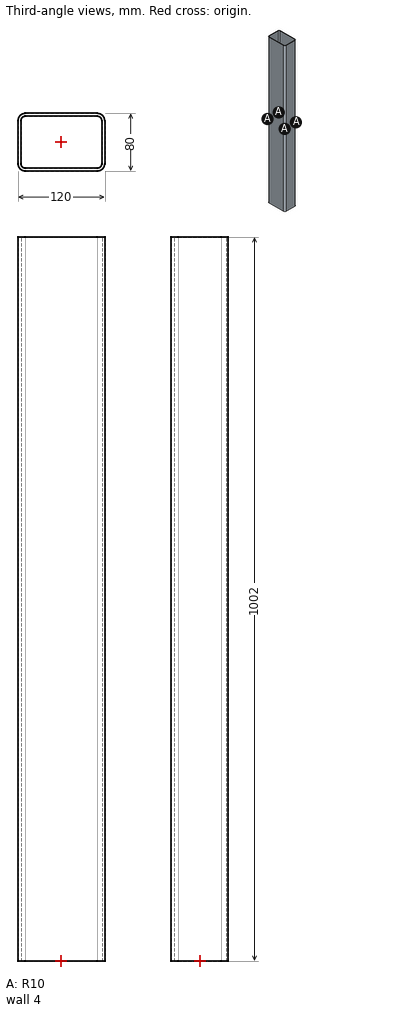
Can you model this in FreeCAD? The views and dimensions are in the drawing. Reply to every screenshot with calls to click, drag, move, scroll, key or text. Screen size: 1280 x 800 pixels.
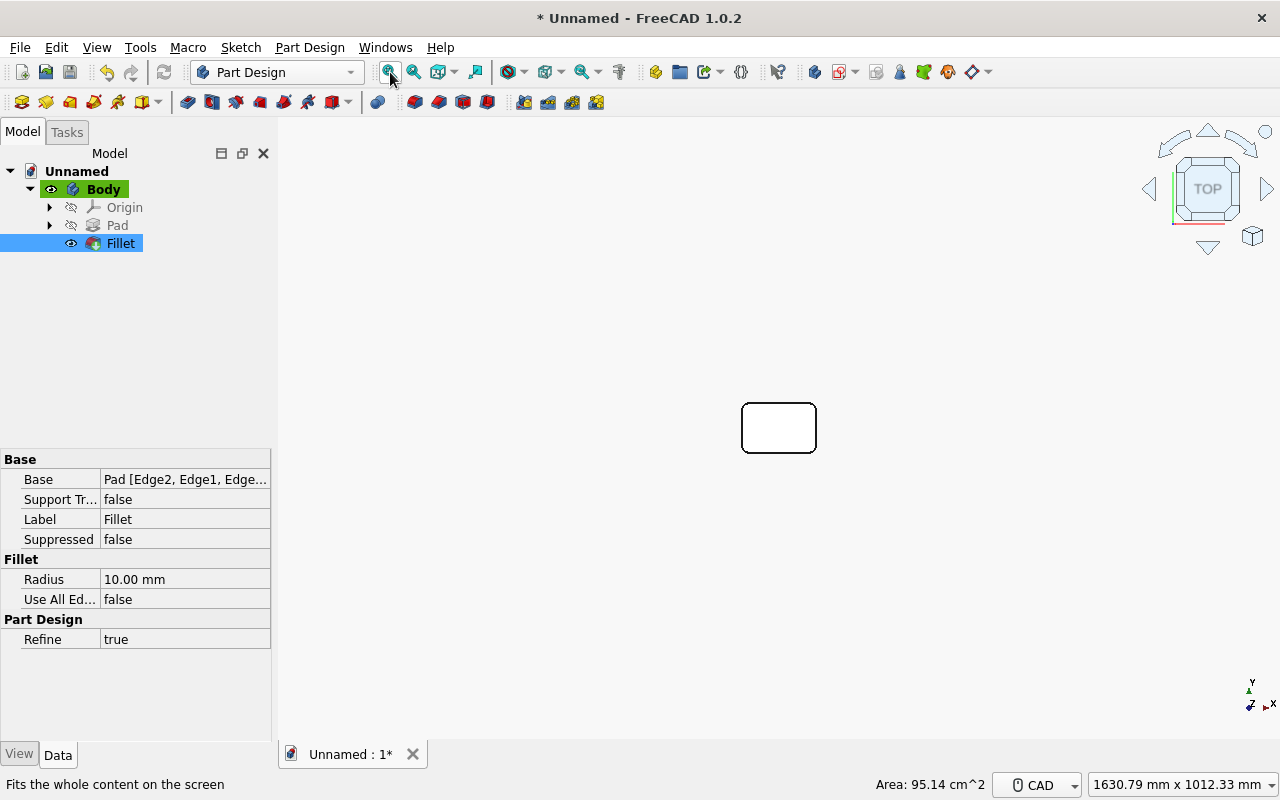
key(1)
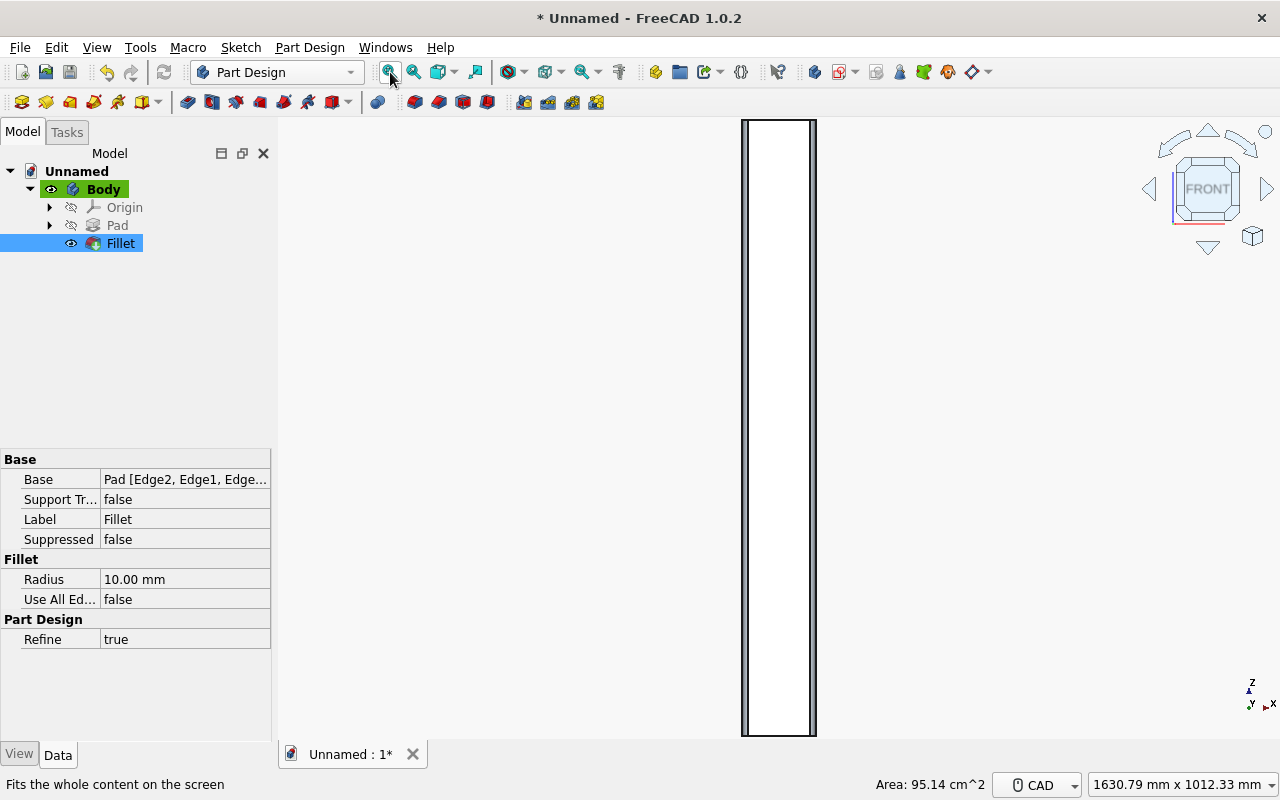
key(3)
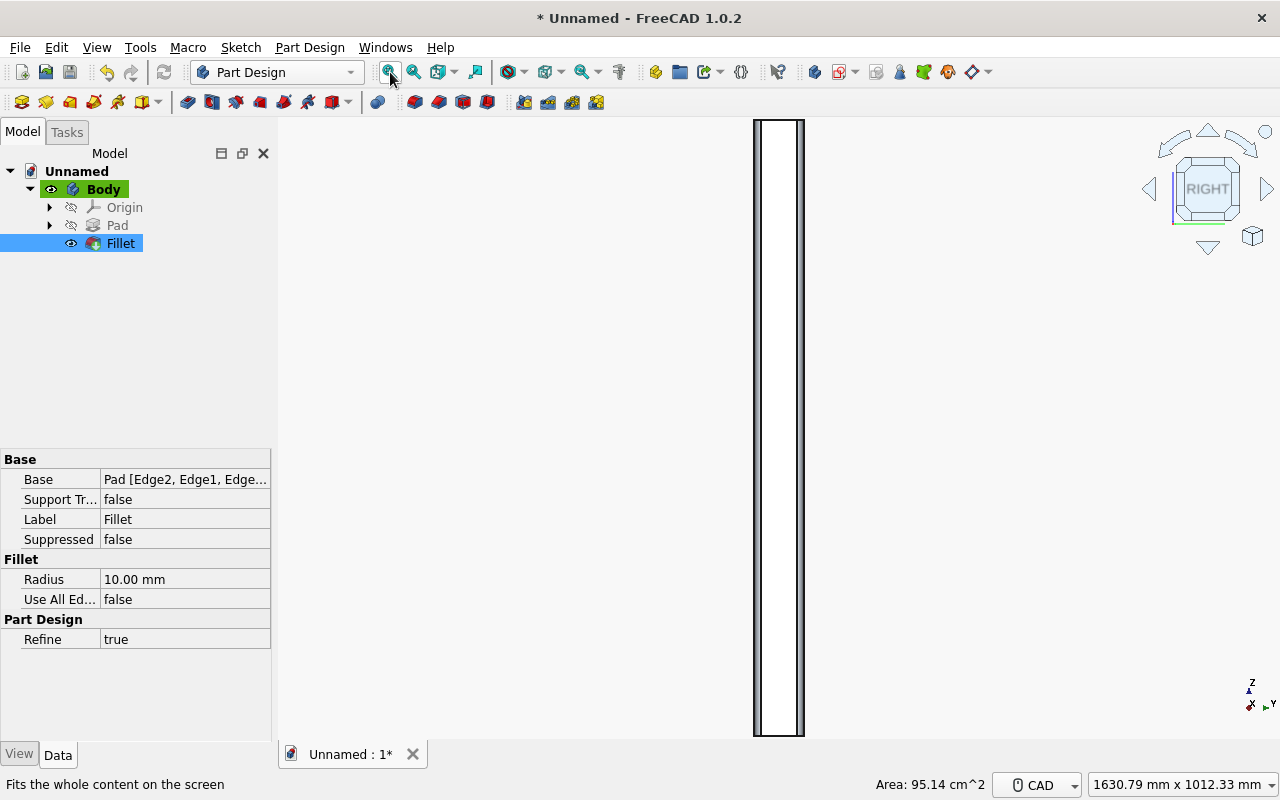
key(5)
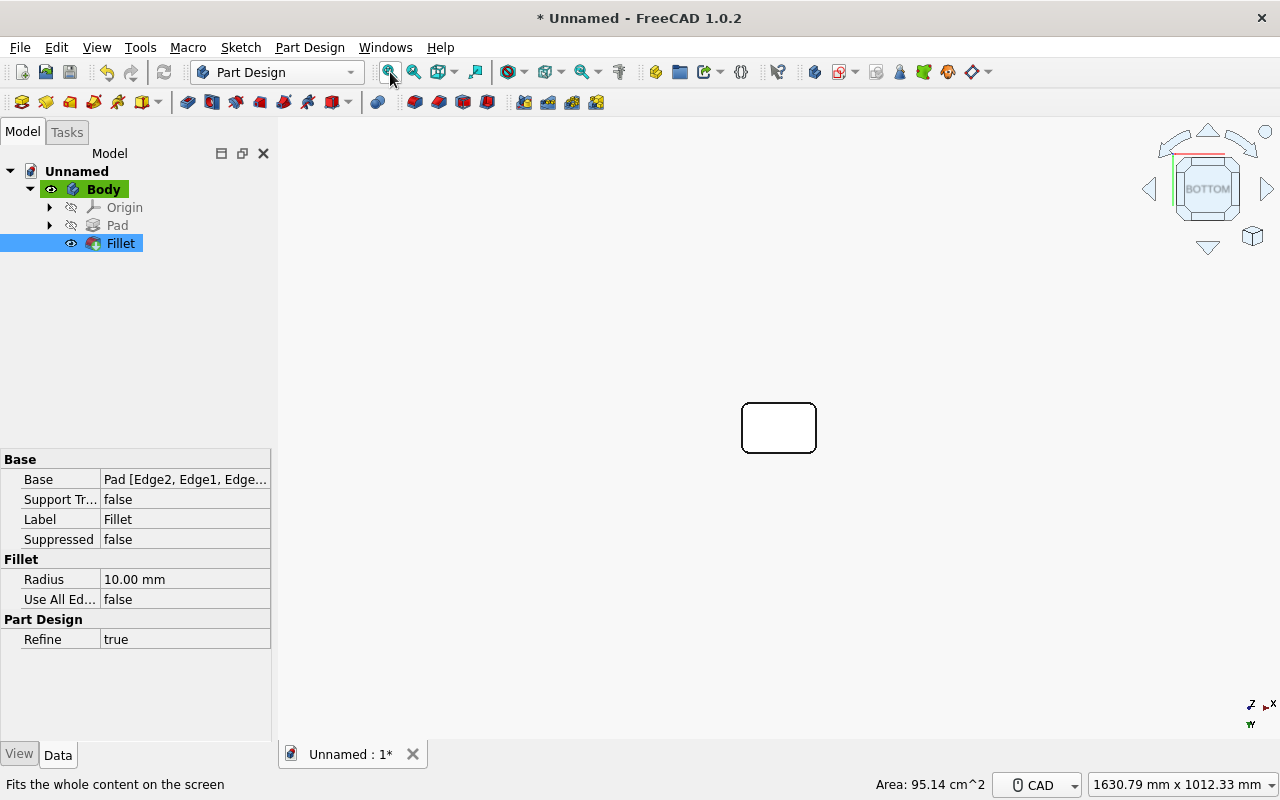
click(390, 72)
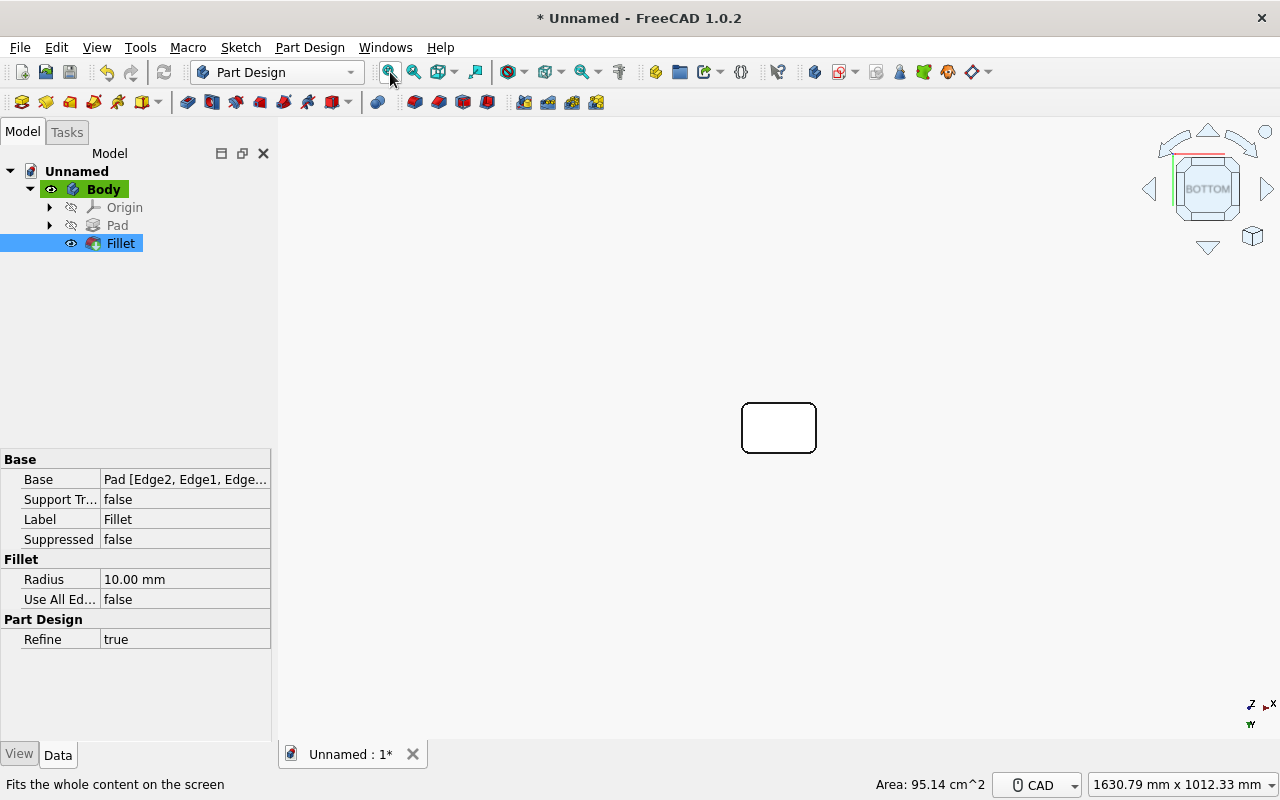
click(790, 427, ctrl)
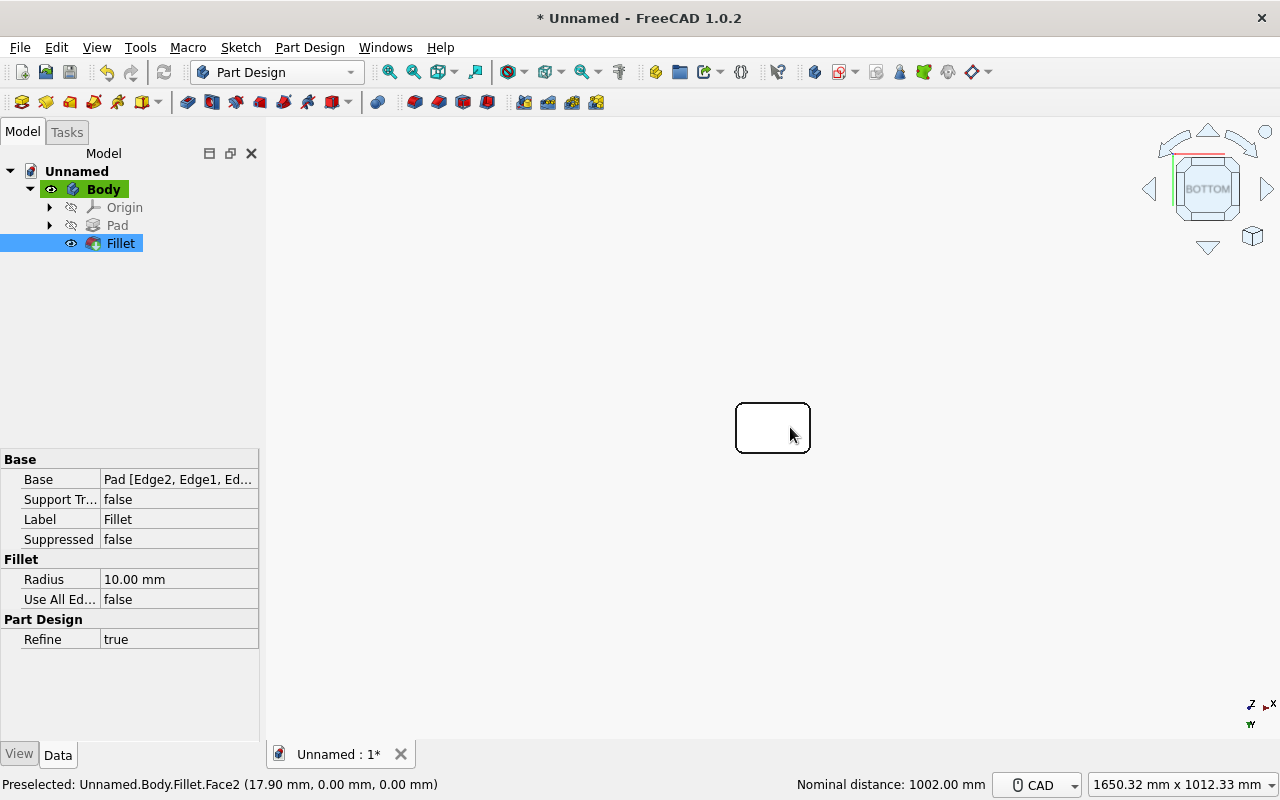
click(488, 102)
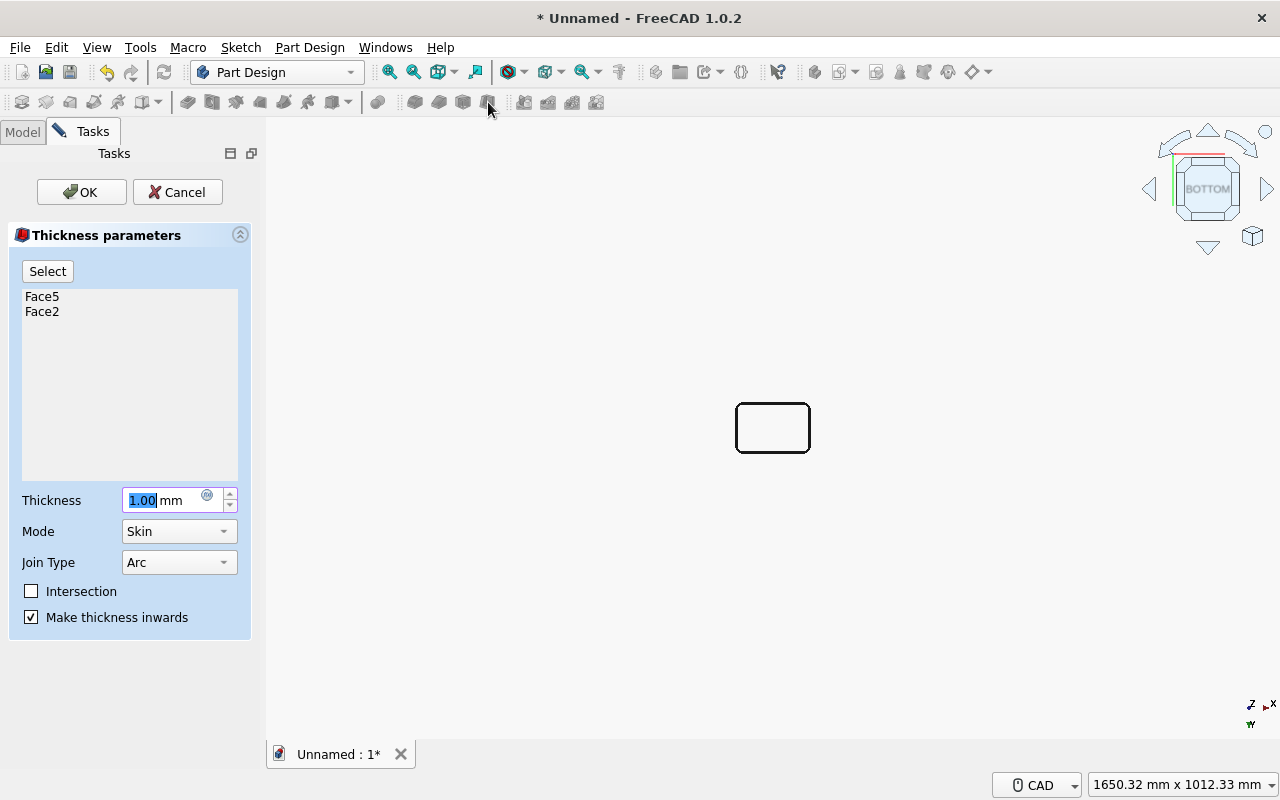
text(4)
key(Tab)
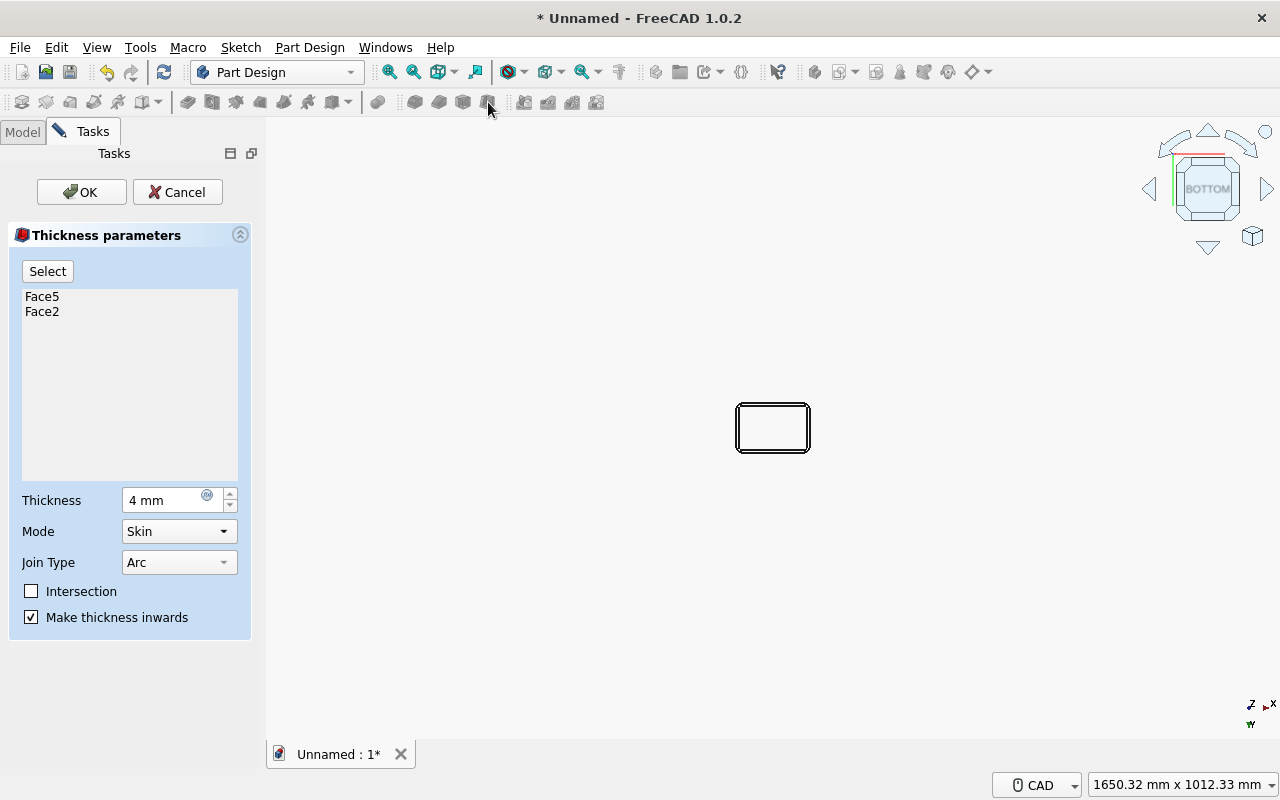
click(180, 562)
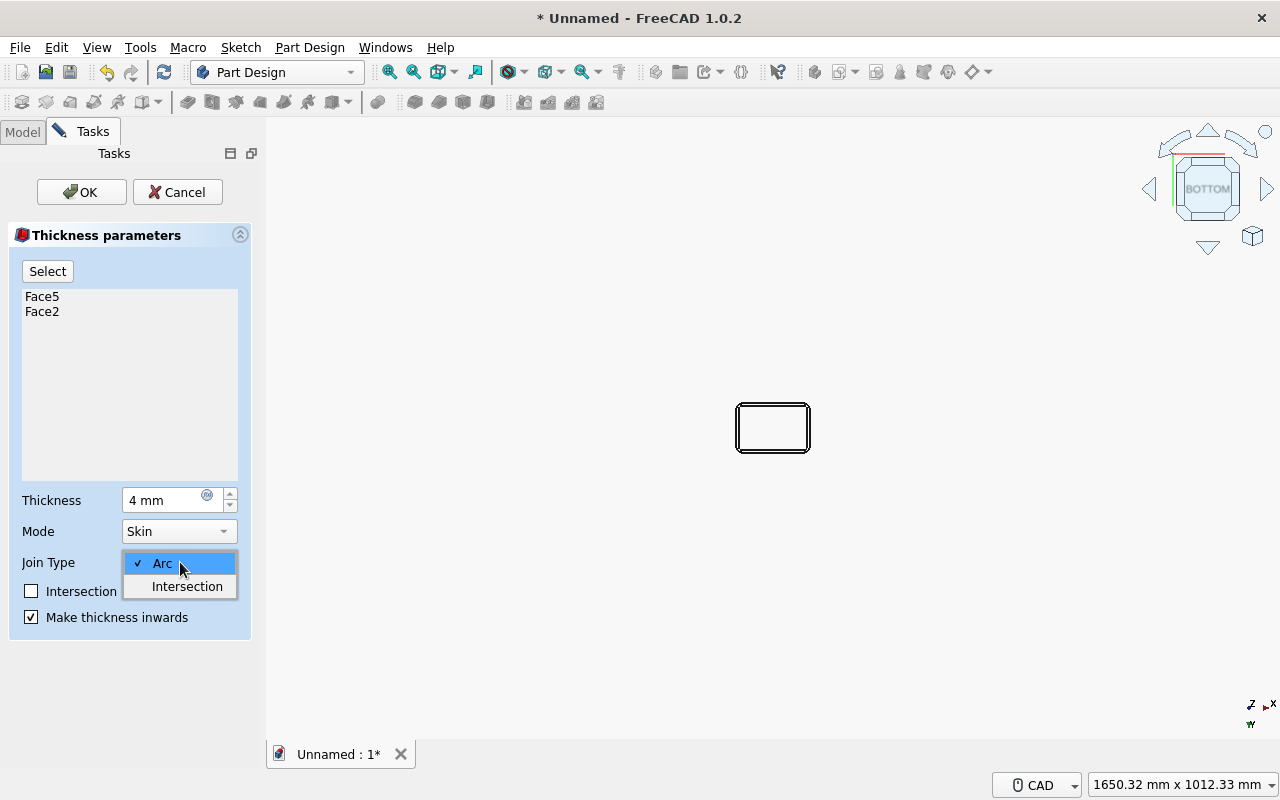
click(179, 586)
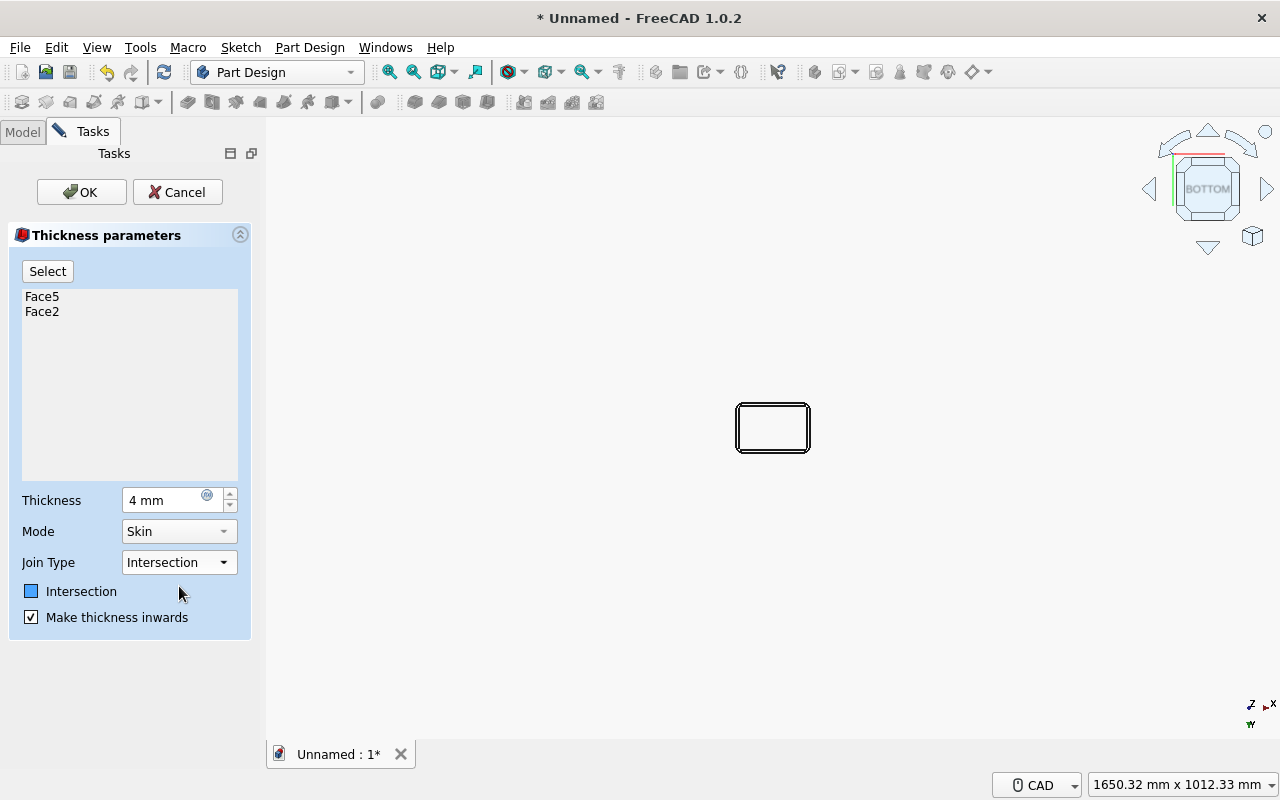
click(82, 192)